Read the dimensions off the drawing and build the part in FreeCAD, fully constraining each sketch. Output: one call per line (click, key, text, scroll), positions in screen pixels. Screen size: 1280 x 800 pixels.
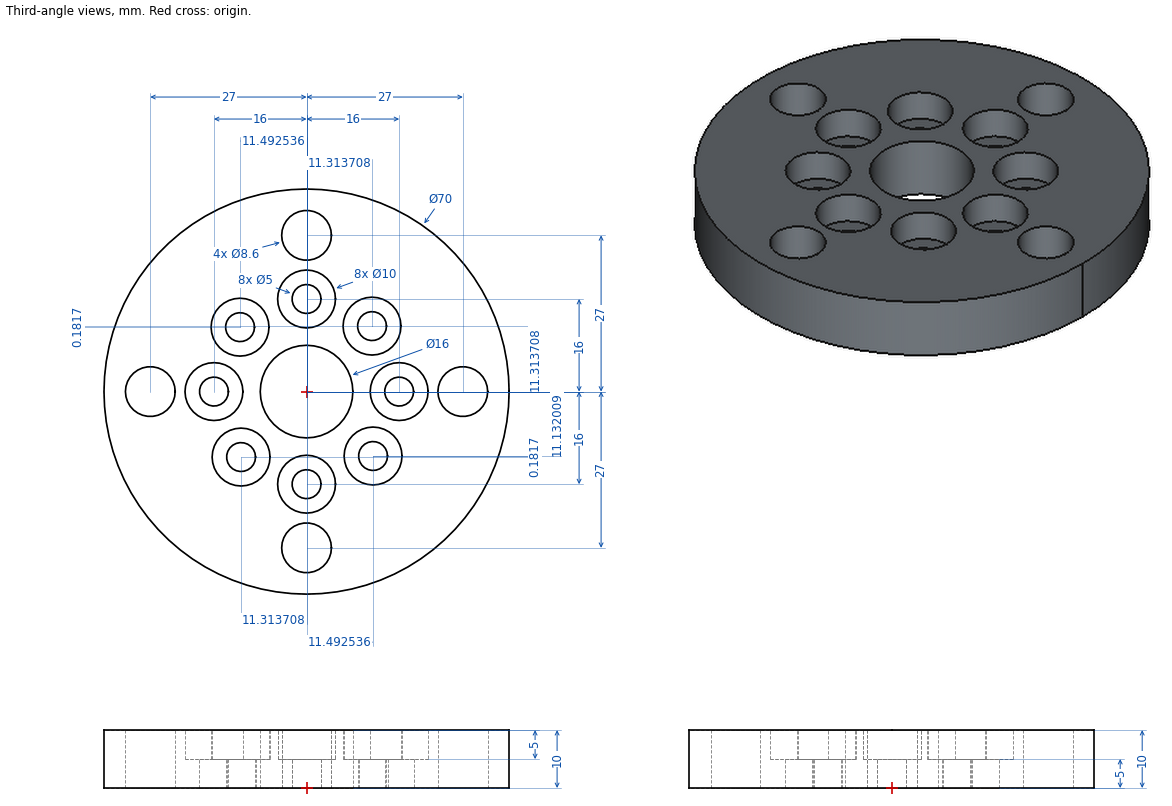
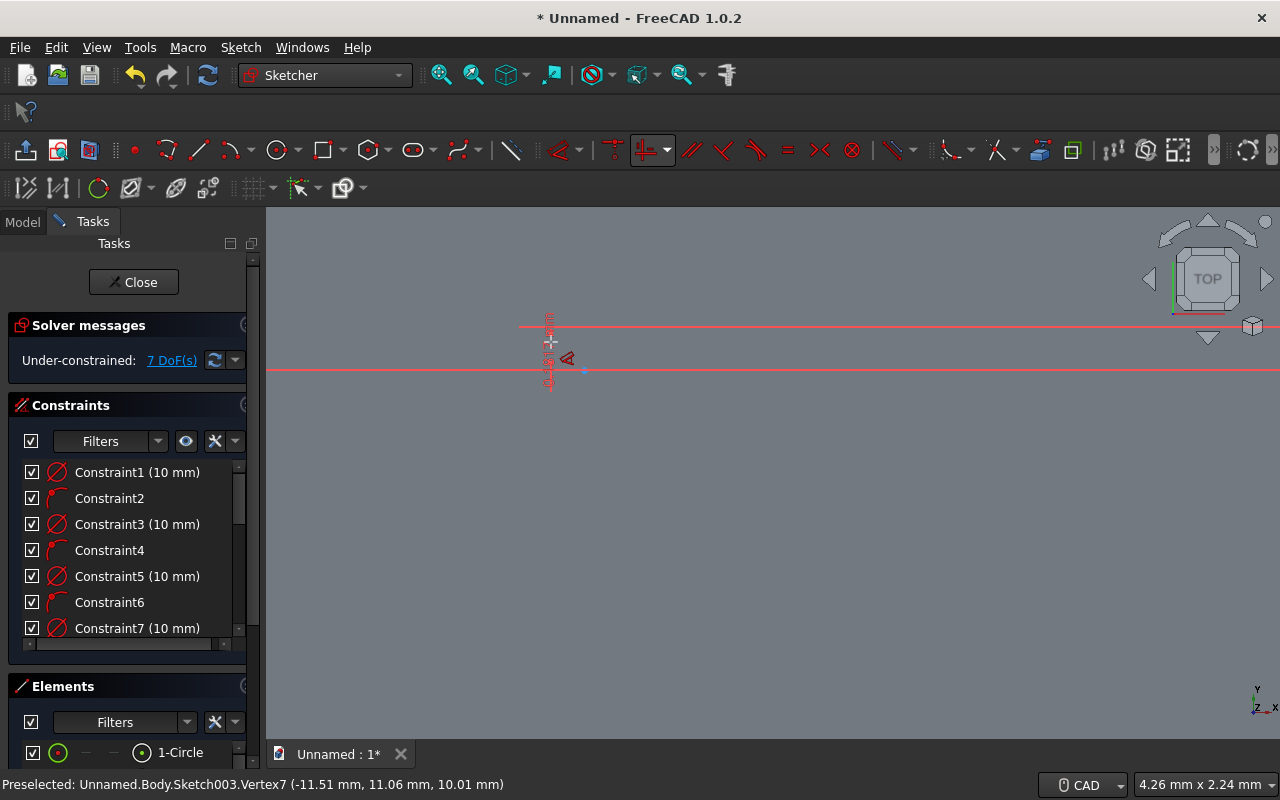
scroll(593, 366, down, 16)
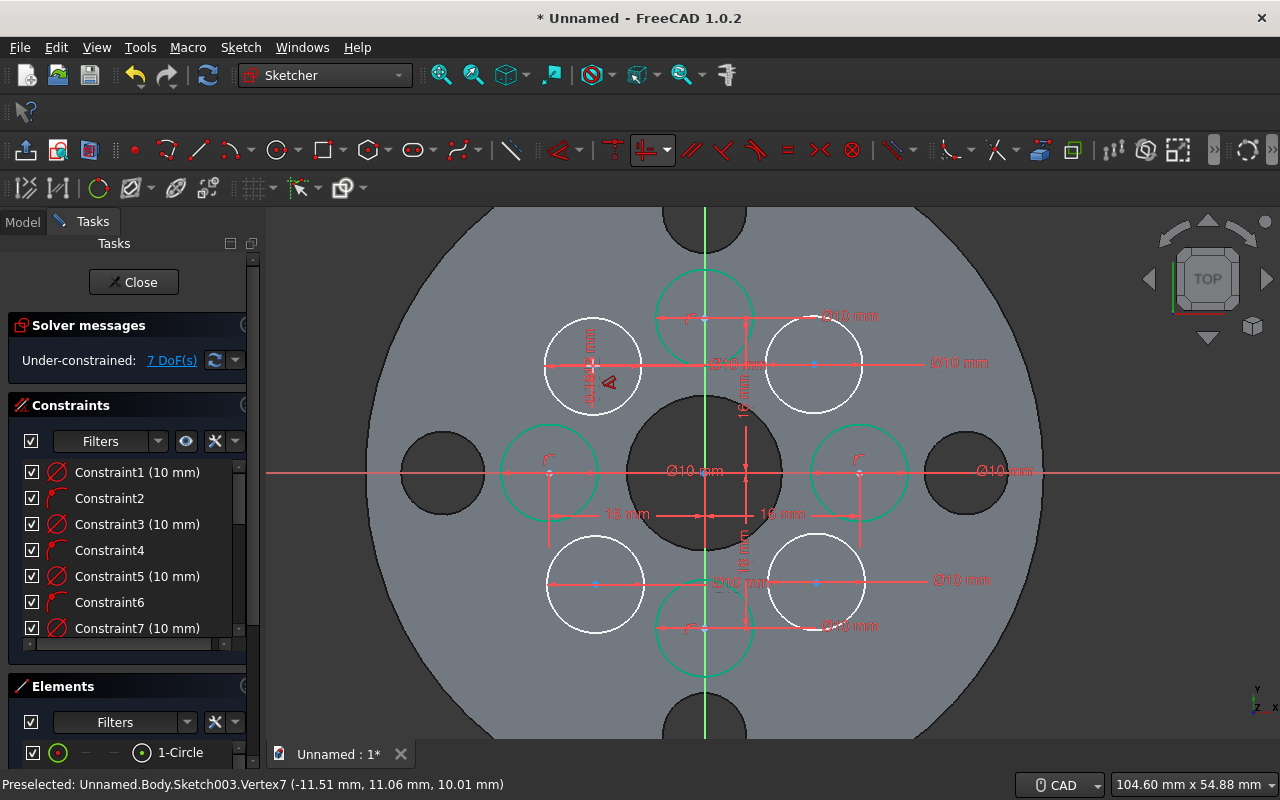
scroll(816, 582, up, 16)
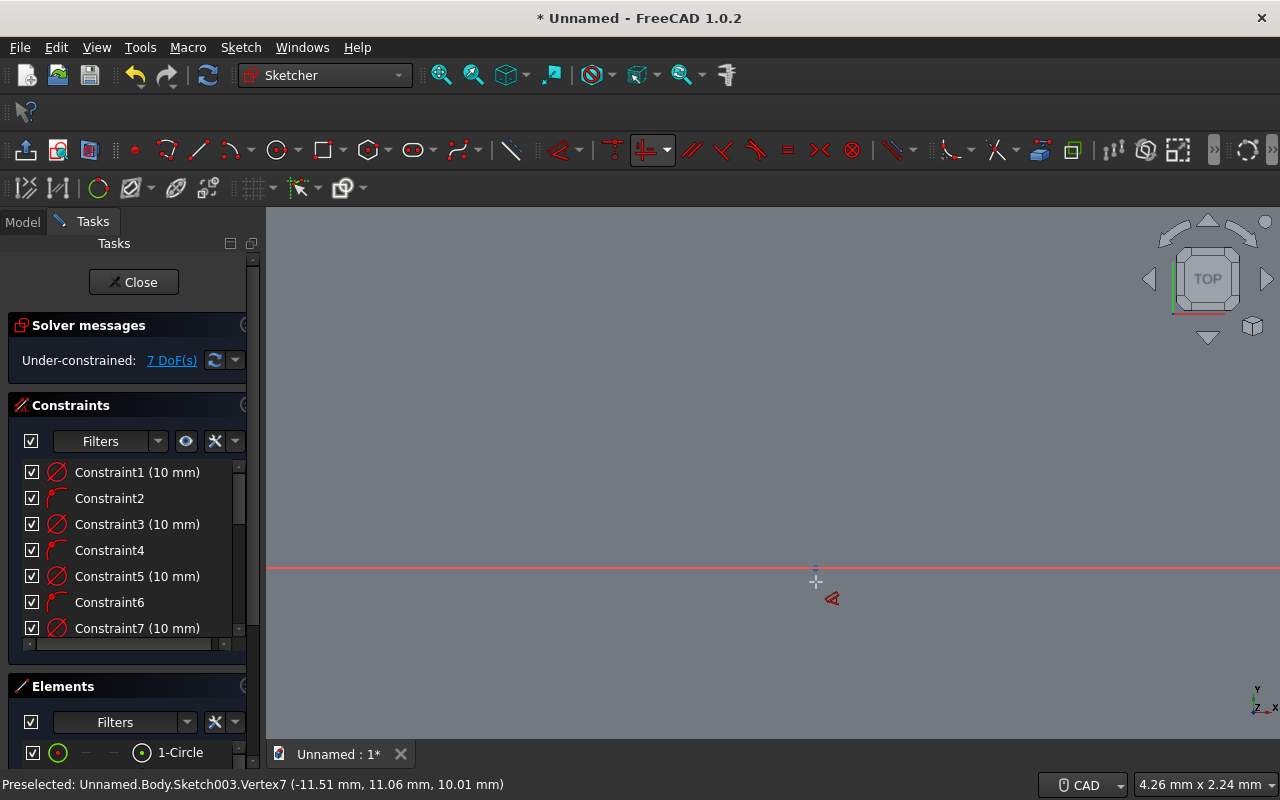
click(815, 568)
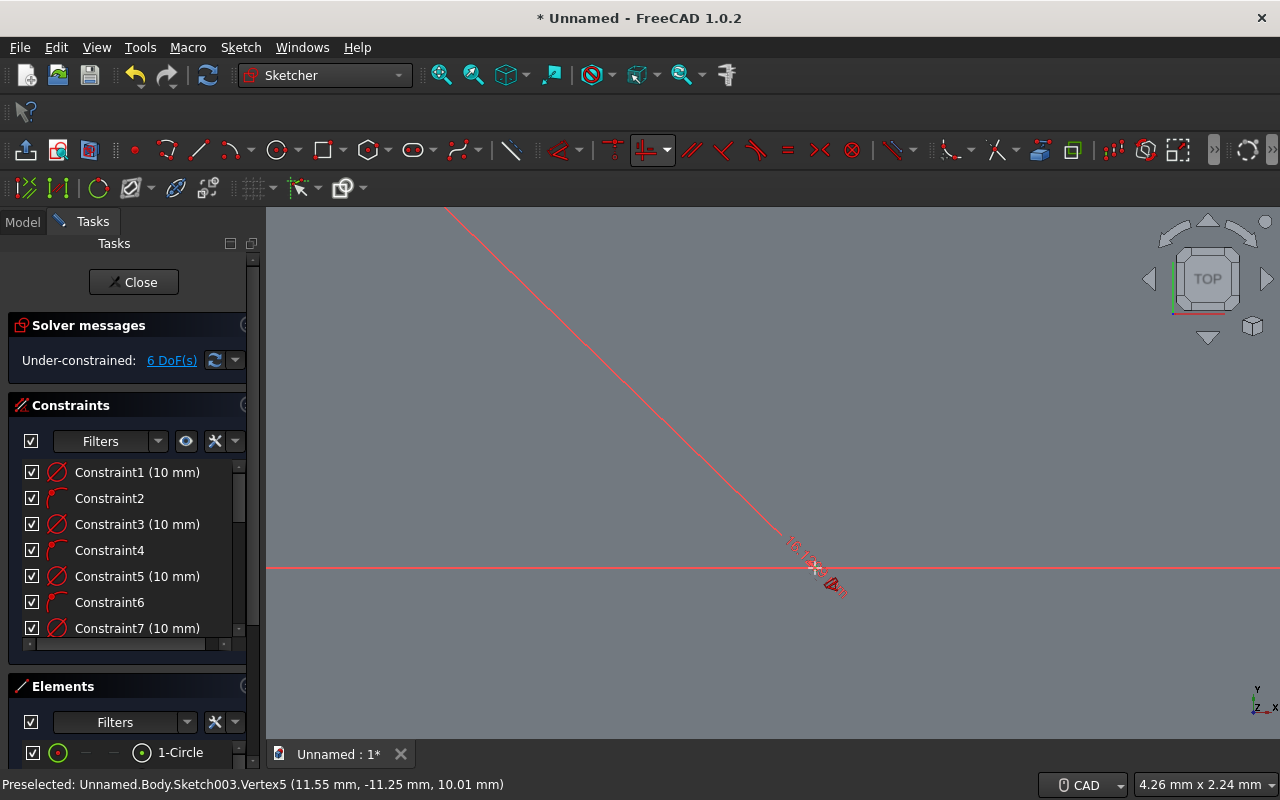
scroll(817, 583, down, 16)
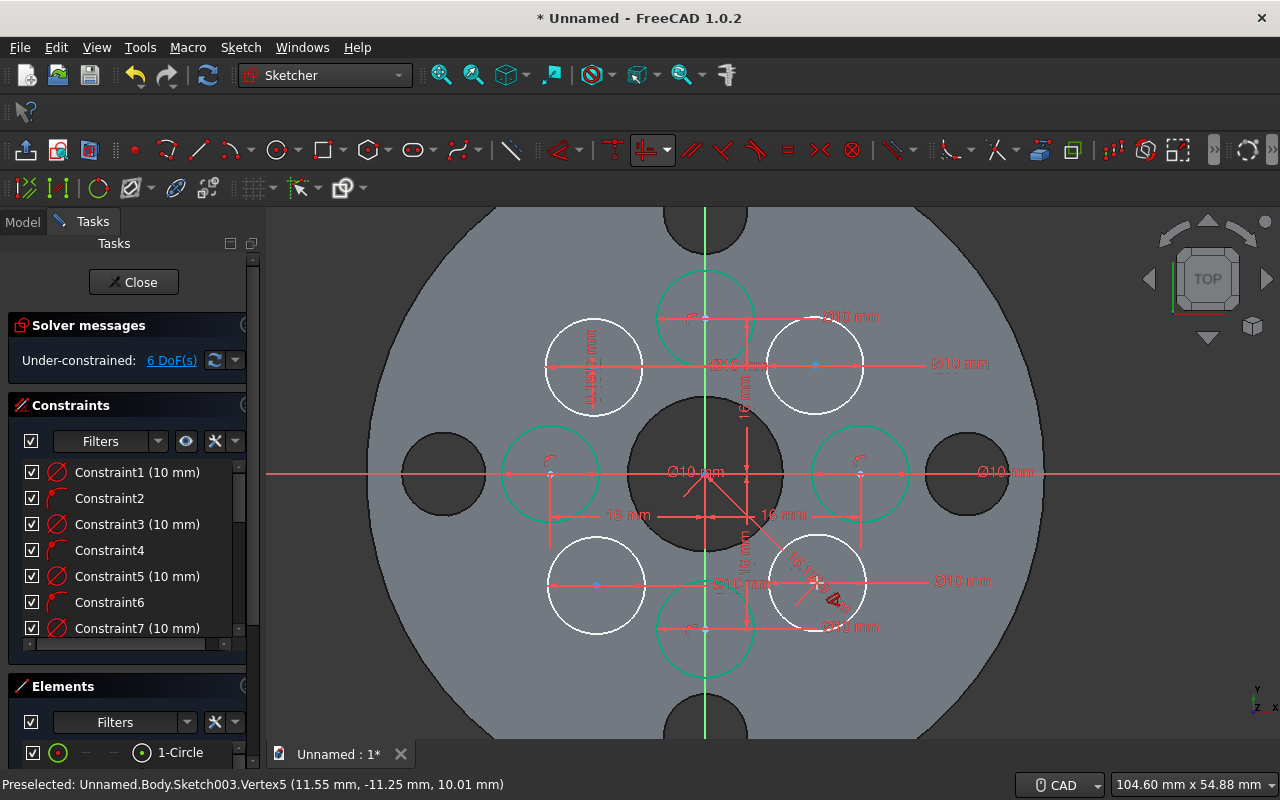
scroll(596, 586, up, 16)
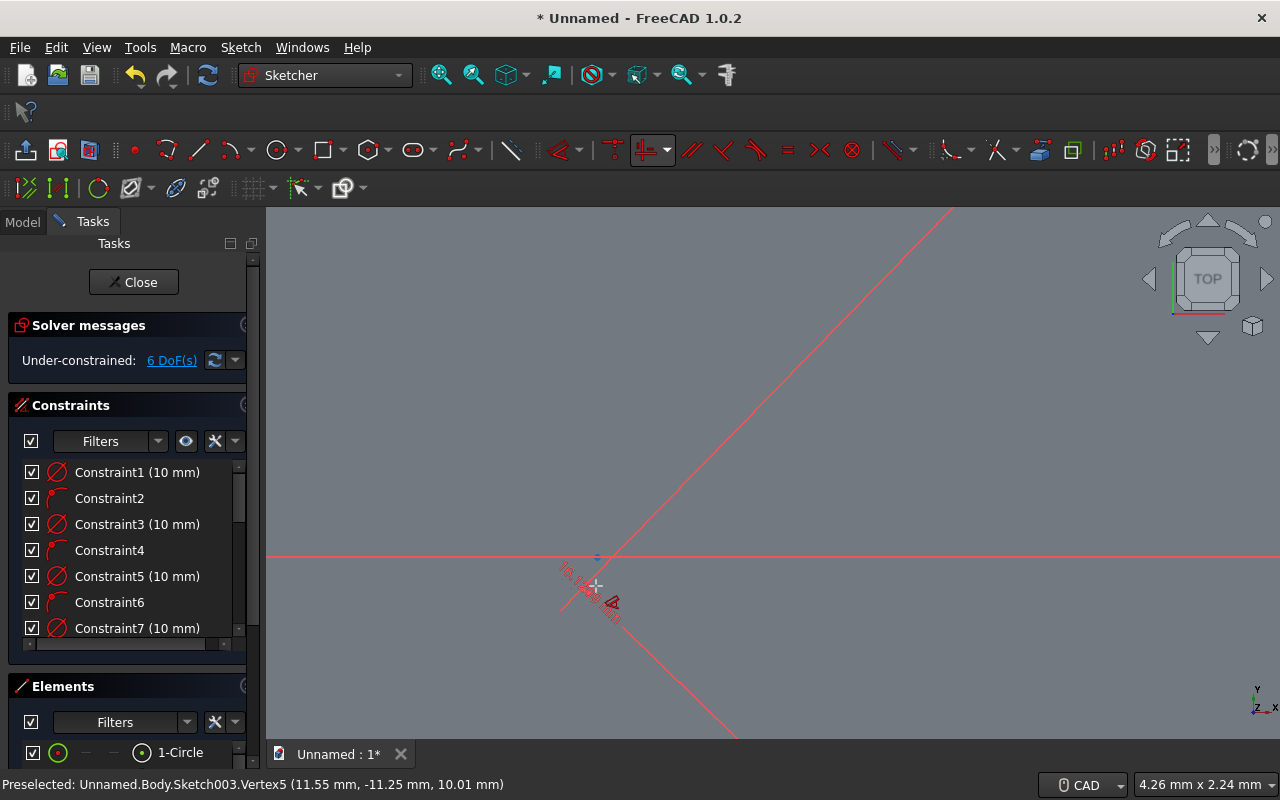
click(598, 557)
click(564, 527)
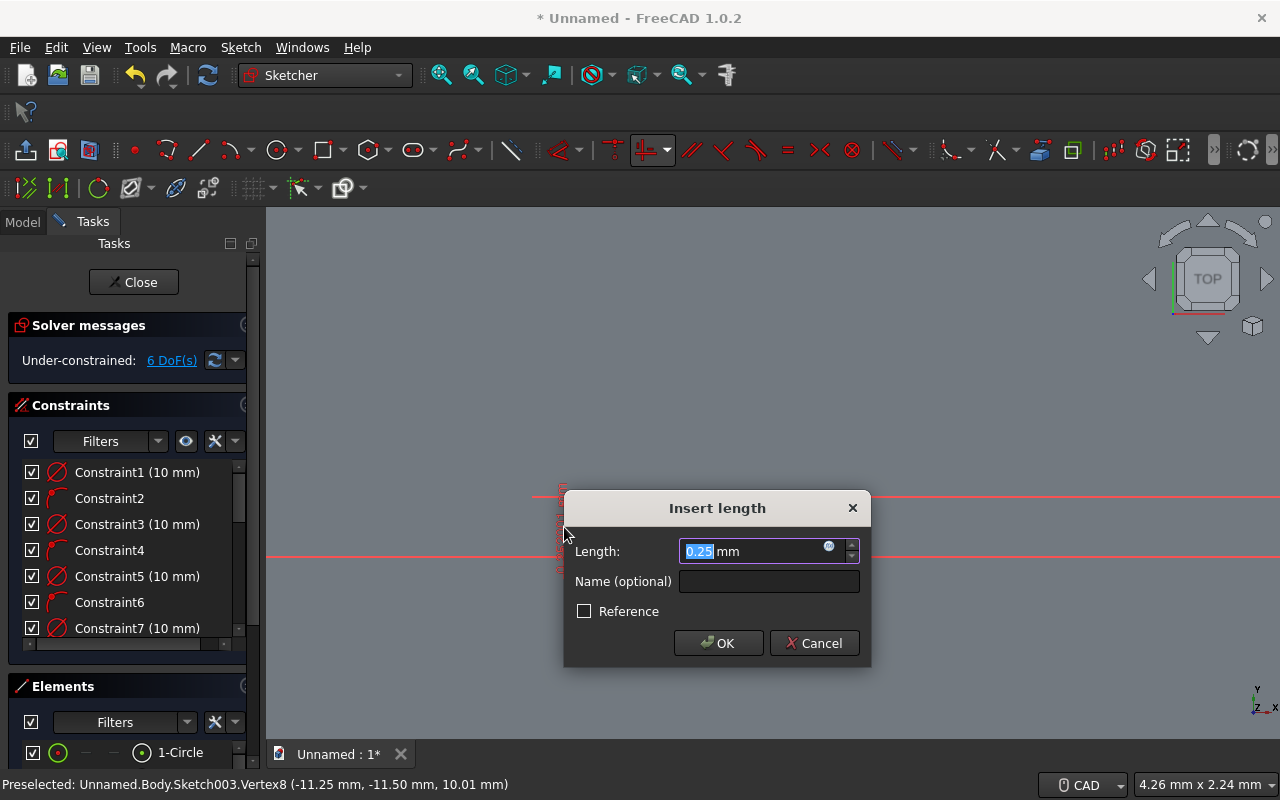
text(0.1817)
key(Return)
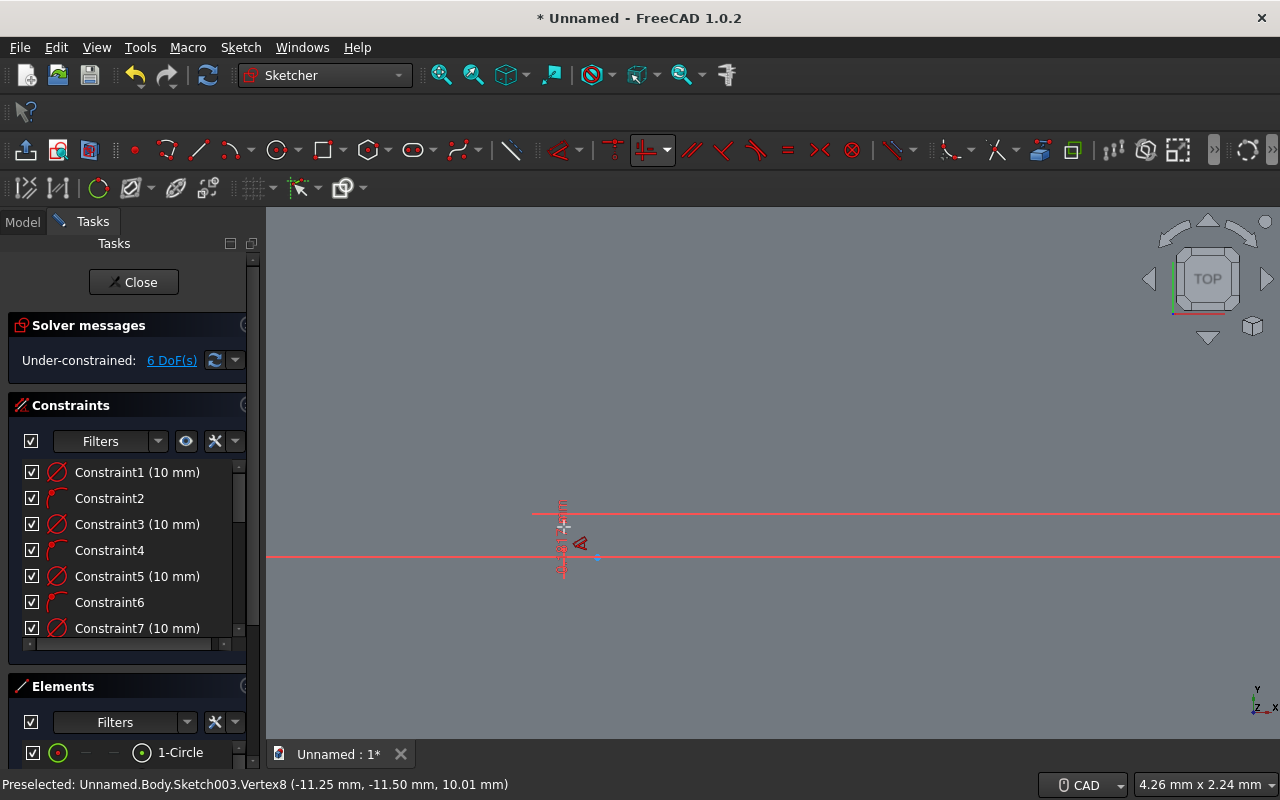
scroll(595, 586, down, 16)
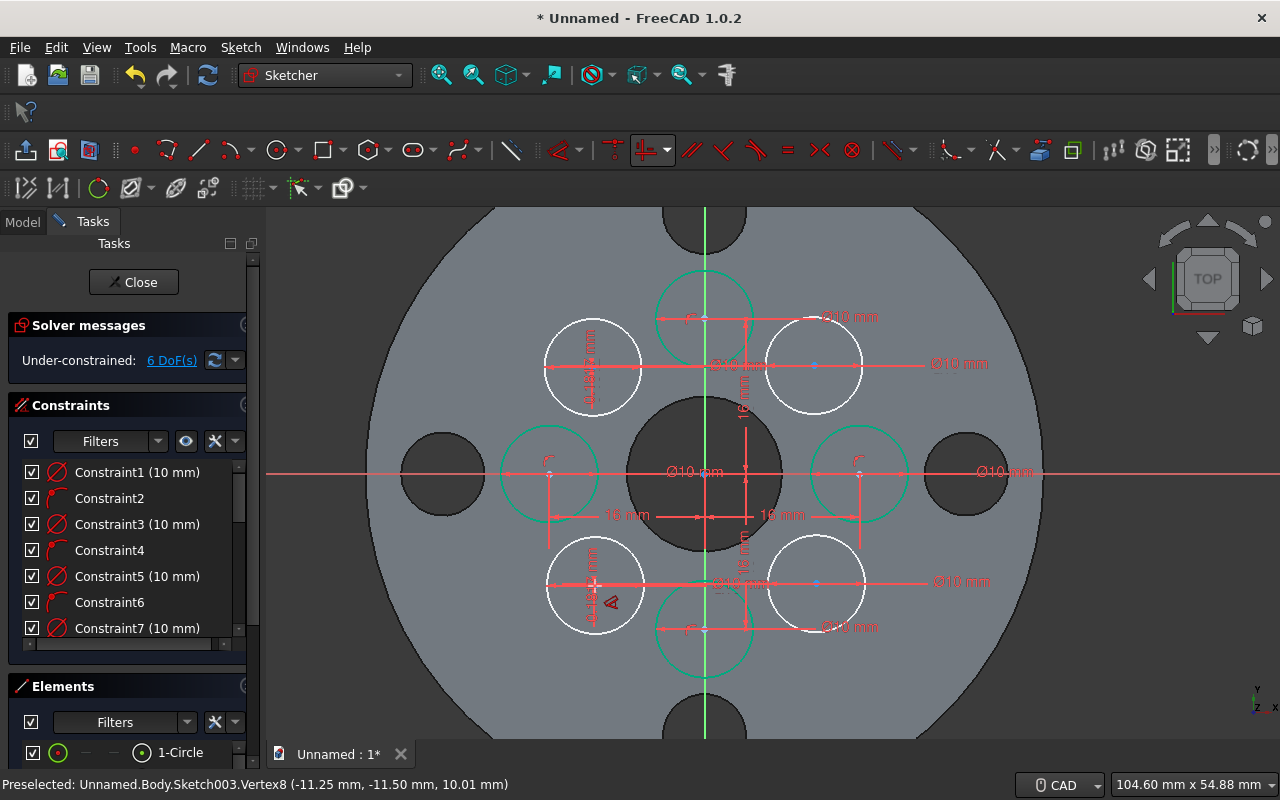
click(816, 584)
click(735, 618)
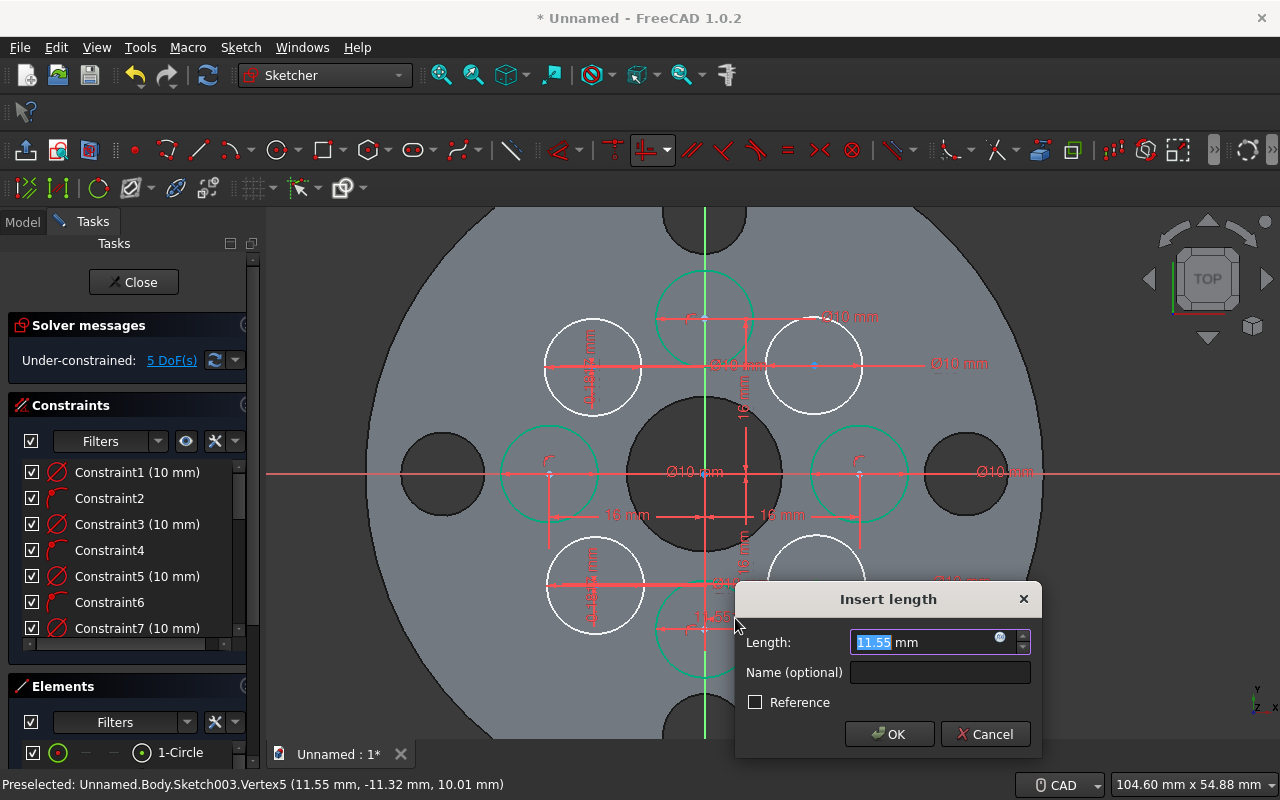
text(11.492536)
key(Return)